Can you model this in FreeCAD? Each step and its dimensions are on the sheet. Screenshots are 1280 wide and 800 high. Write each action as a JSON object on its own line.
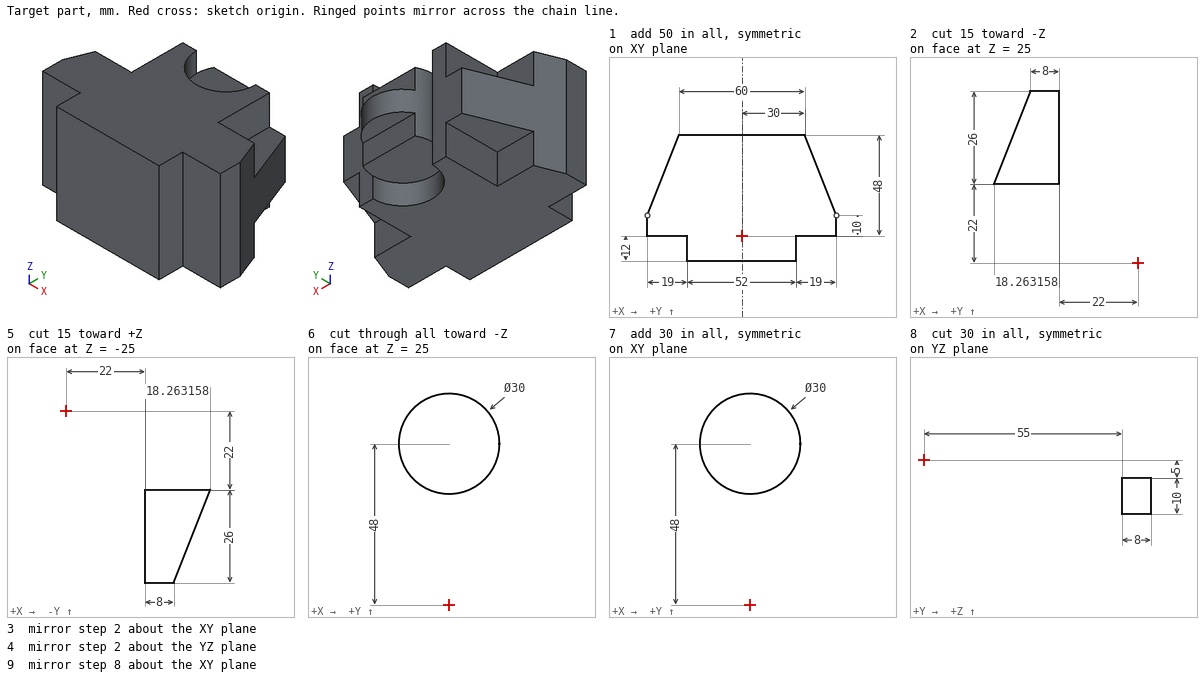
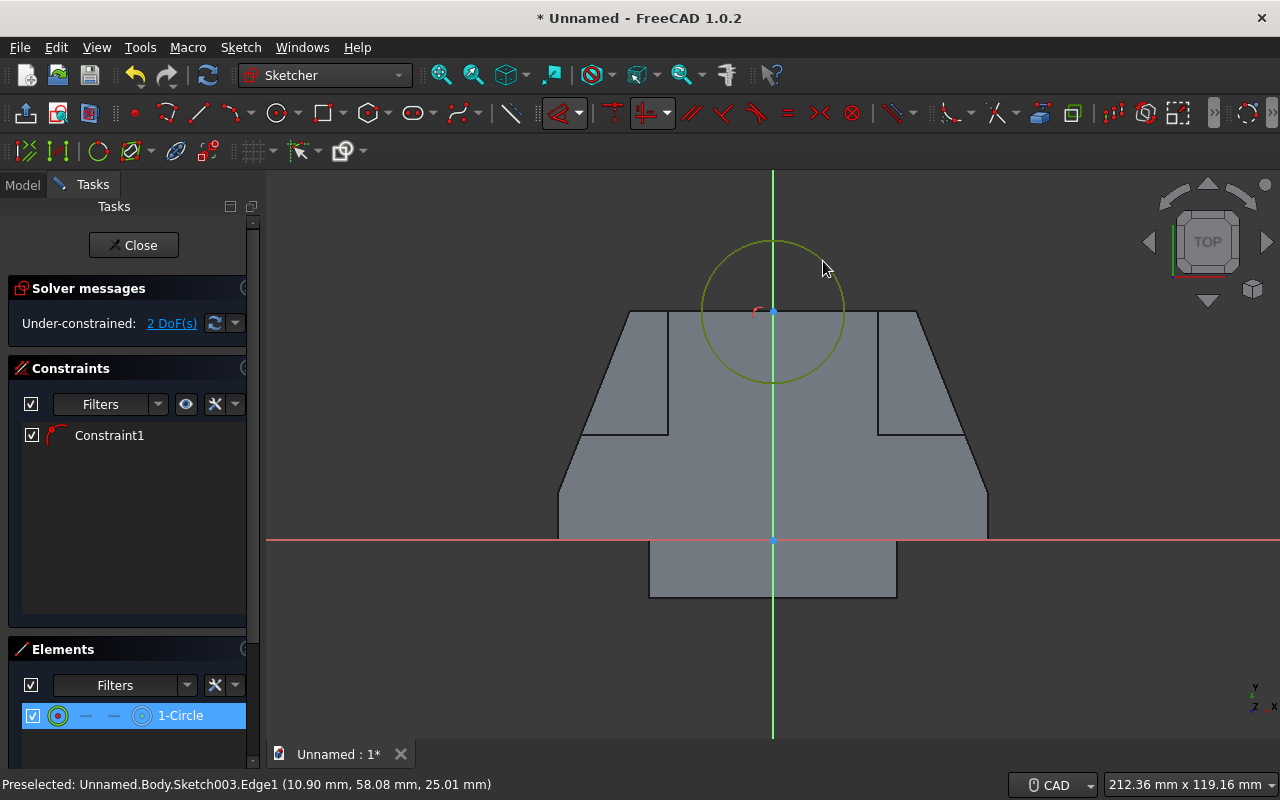
{"action": "left_click", "coordinate": [582, 114]}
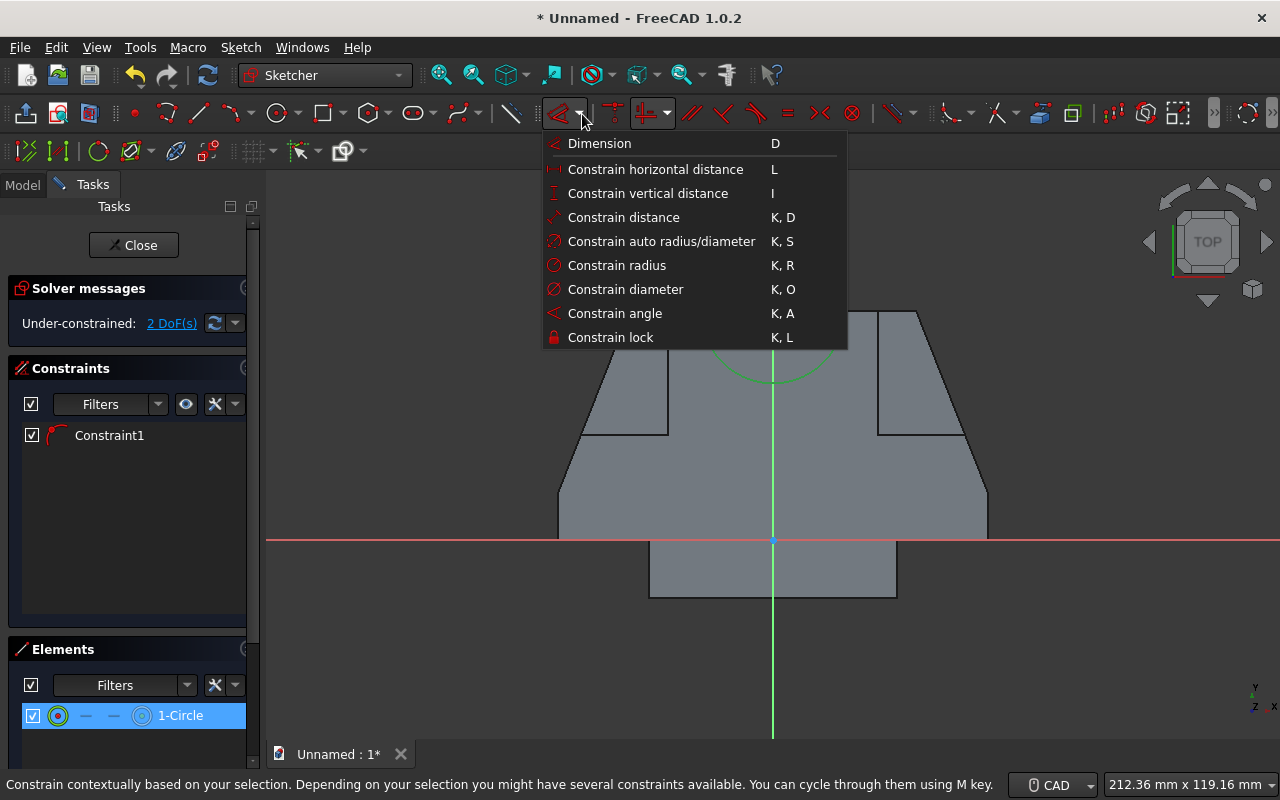
{"action": "left_click", "coordinate": [695, 289]}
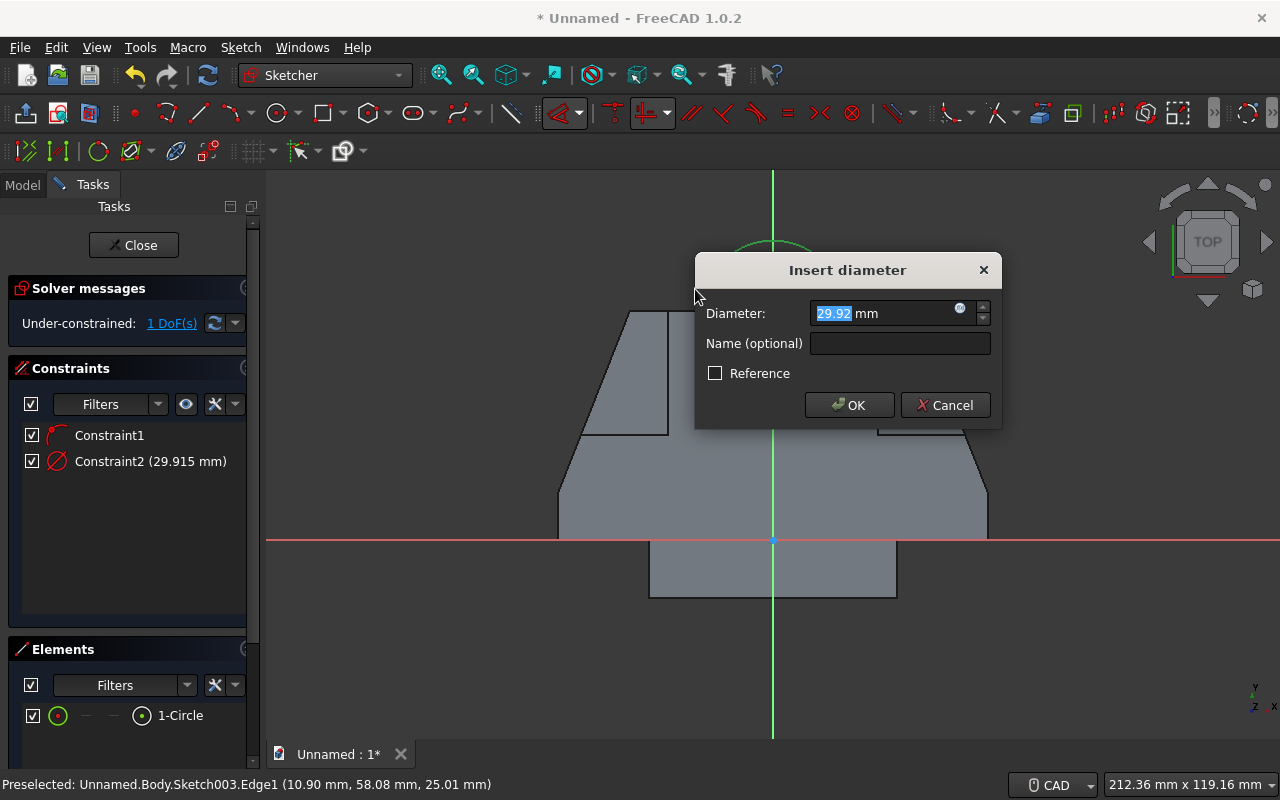
{"action": "type", "text": "30"}
{"action": "key", "text": "Return"}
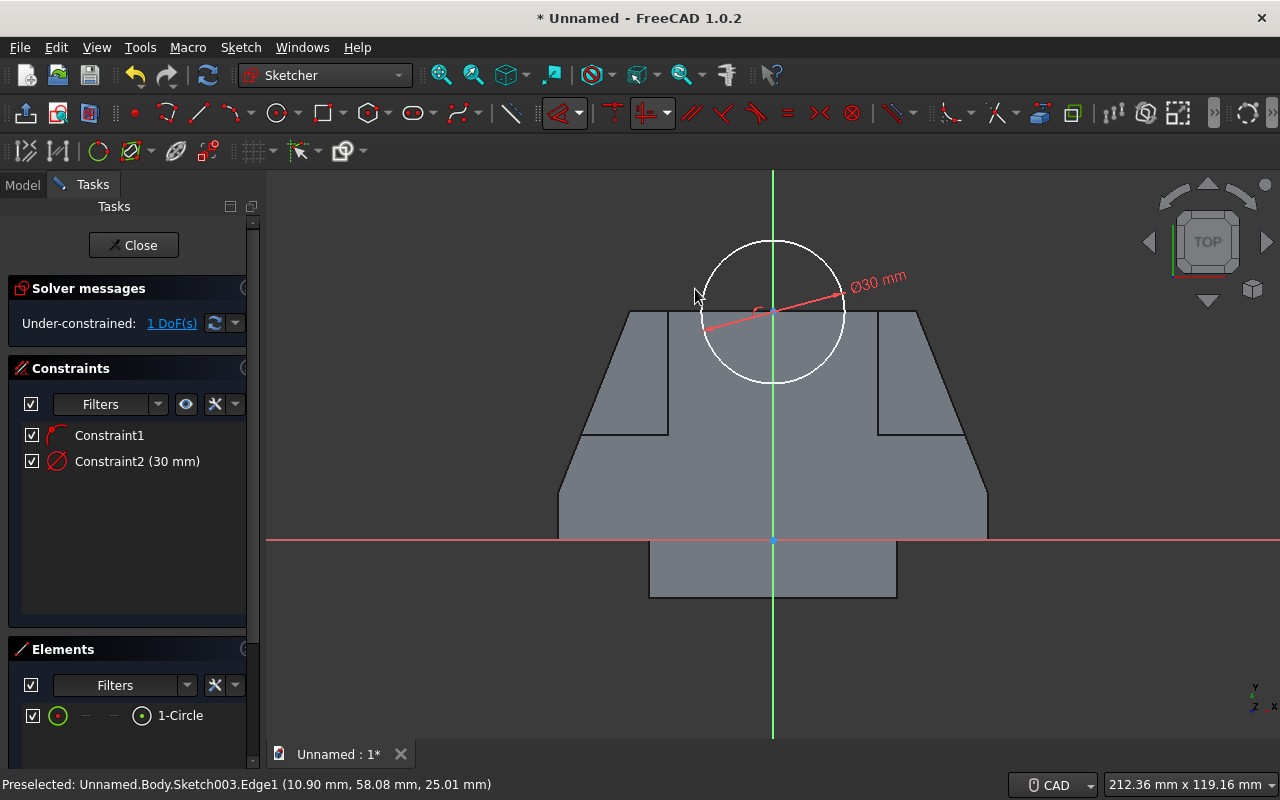
{"action": "left_click", "coordinate": [773, 312]}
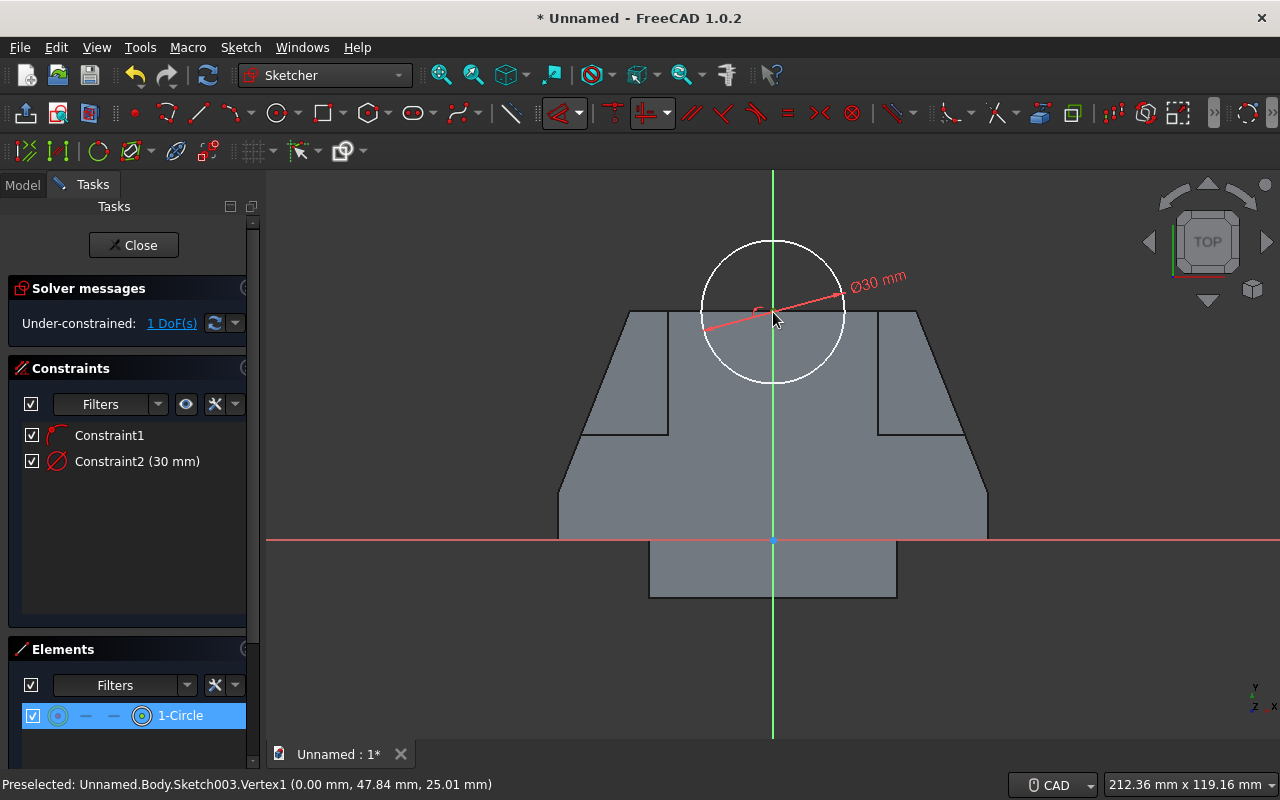
{"action": "left_click", "coordinate": [582, 114]}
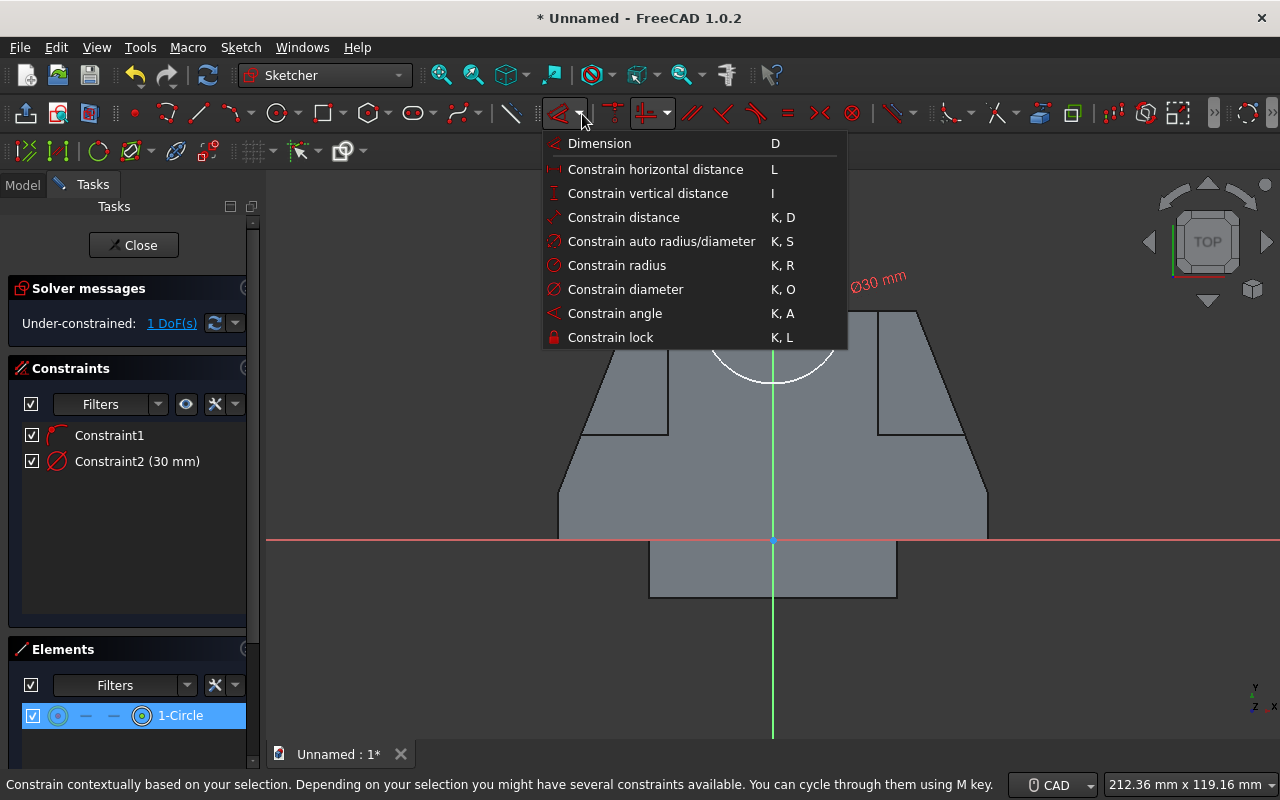
{"action": "left_click", "coordinate": [695, 193]}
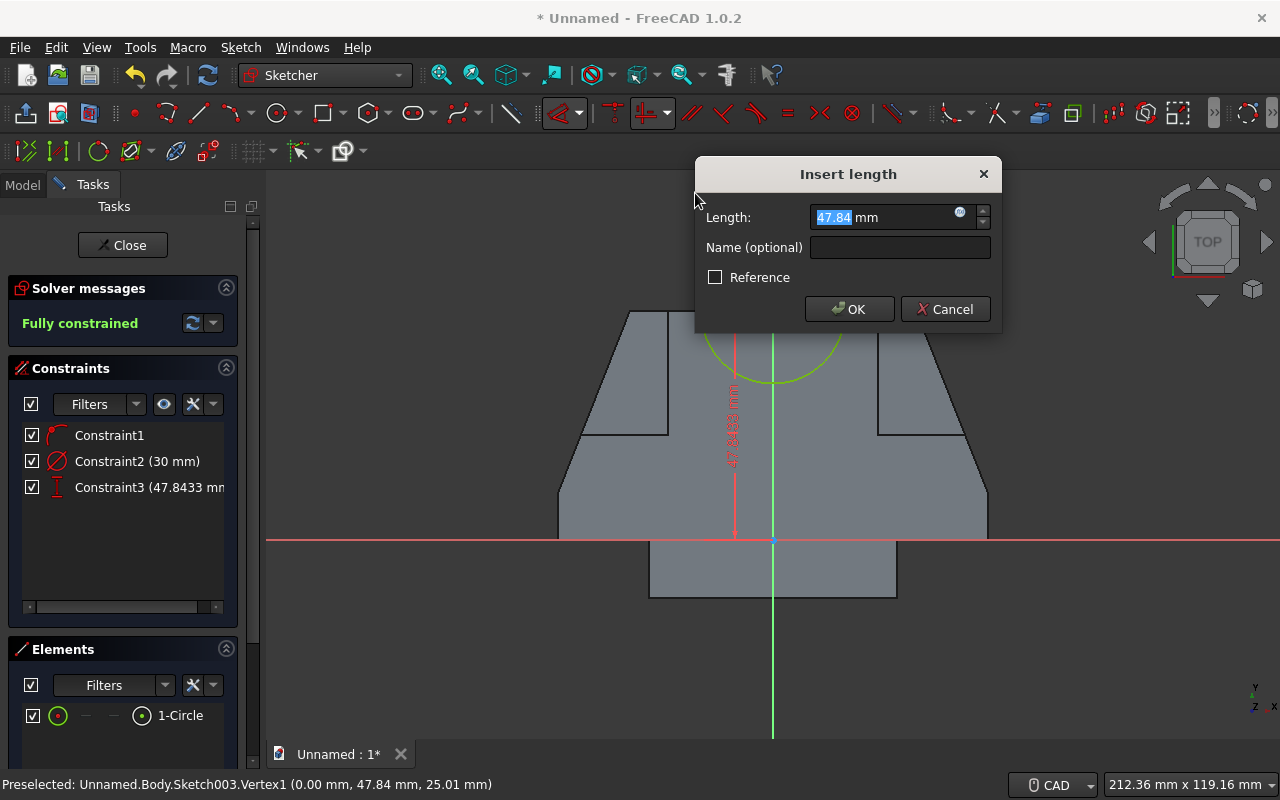
{"action": "type", "text": "48"}
{"action": "key", "text": "Return"}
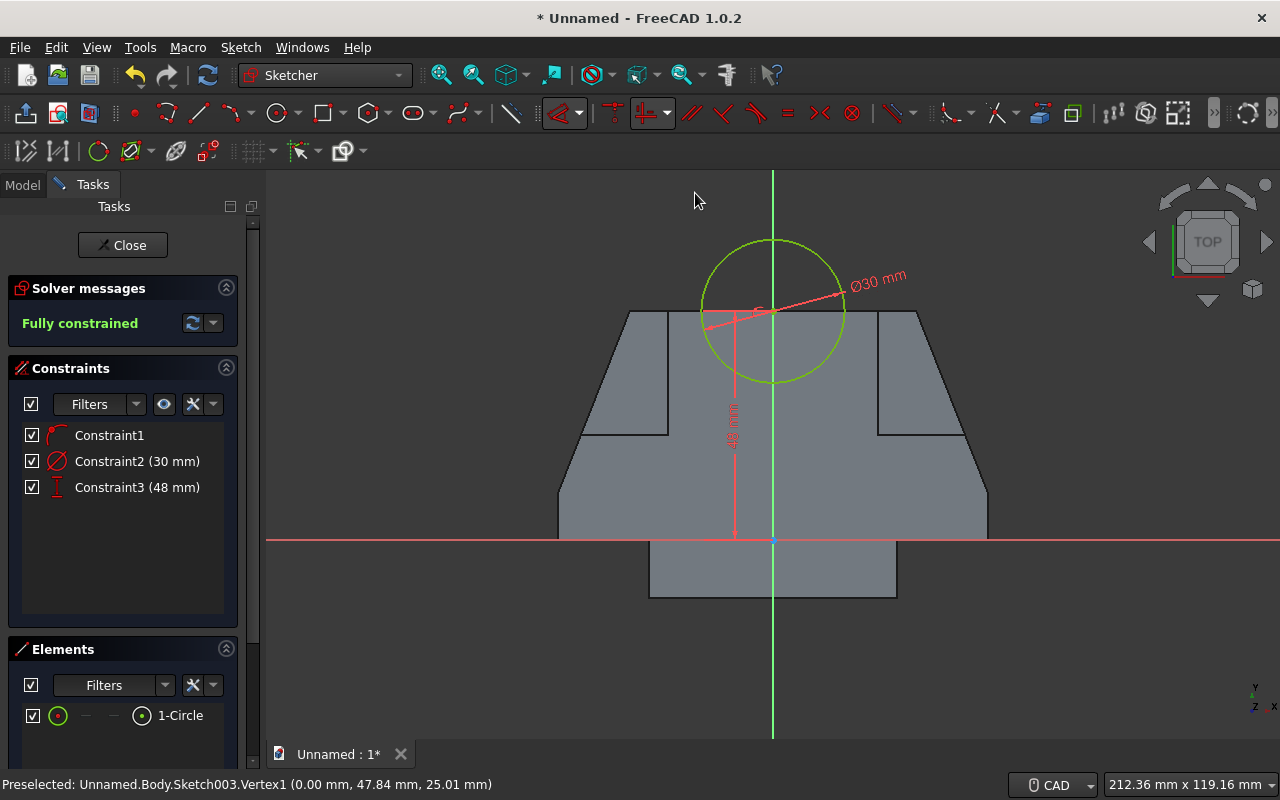
{"action": "left_click", "coordinate": [123, 245]}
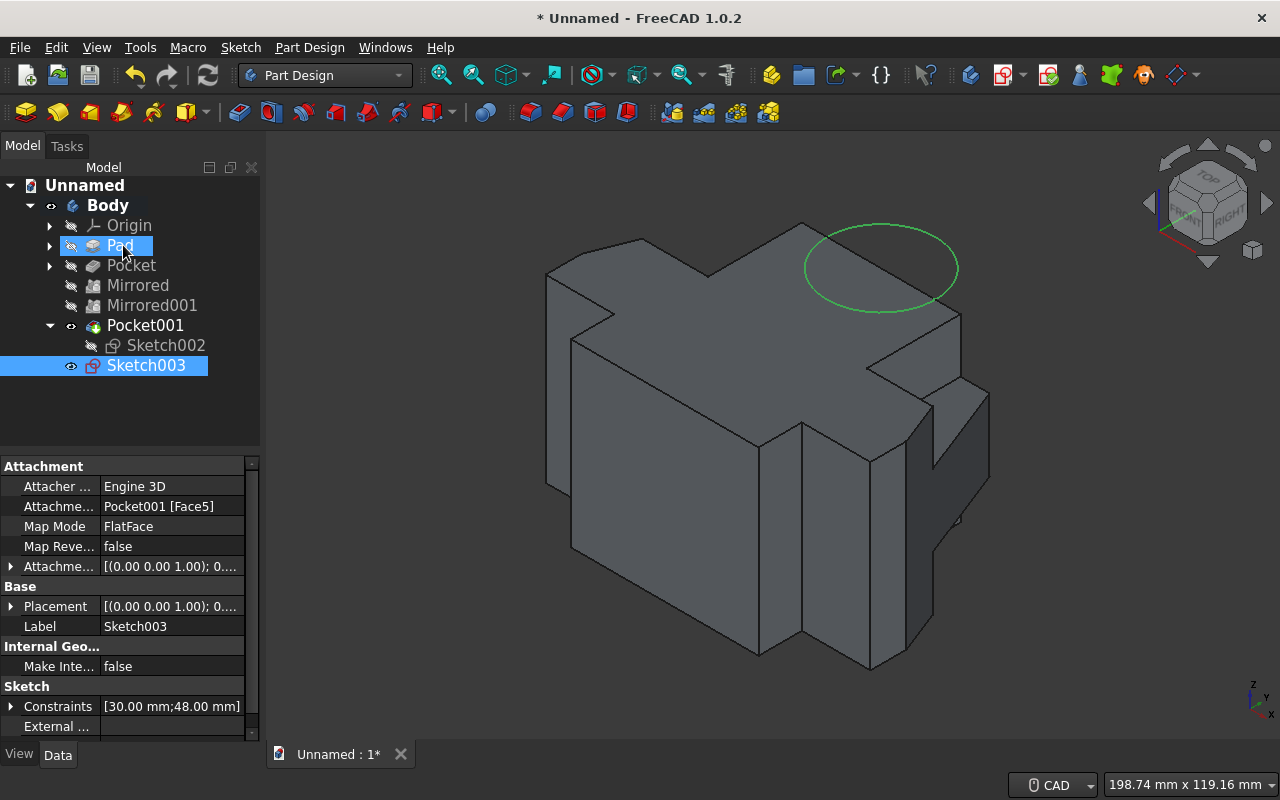
{"action": "left_click", "coordinate": [240, 112]}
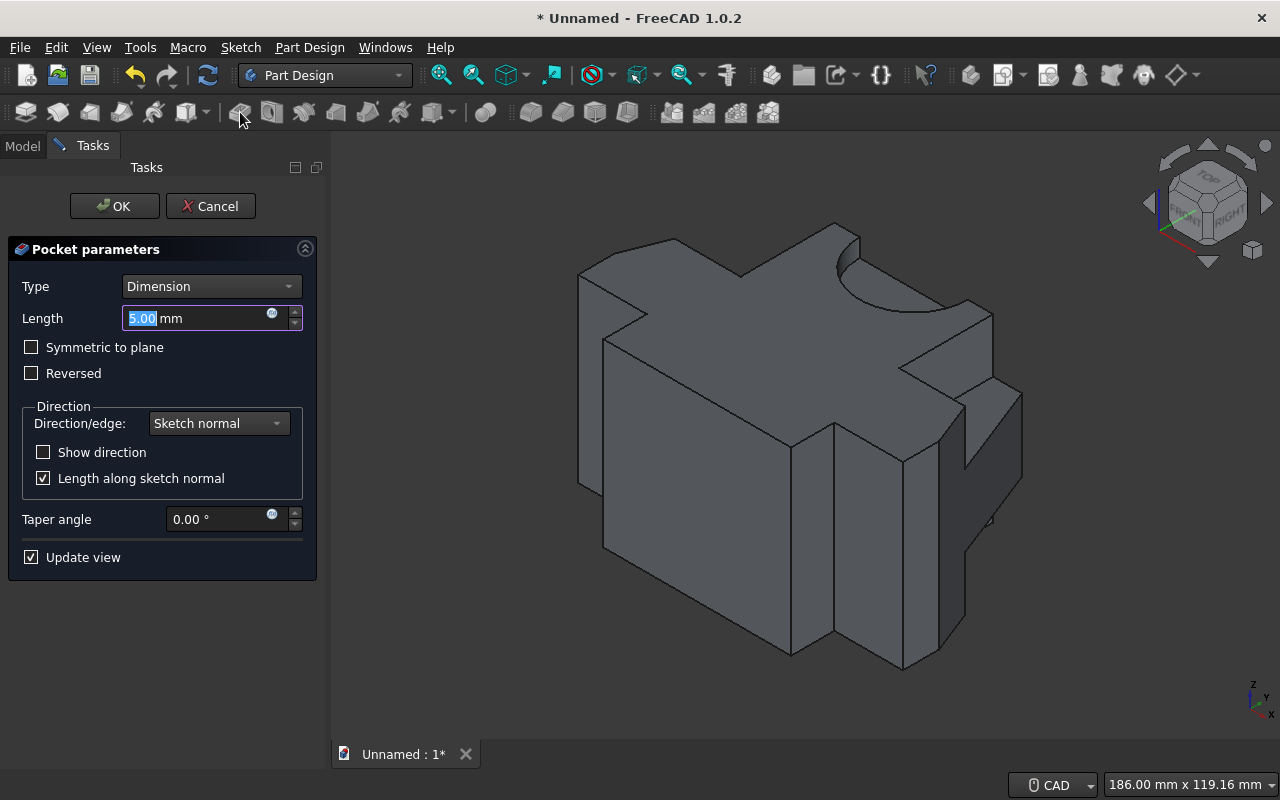
{"action": "left_click", "coordinate": [212, 286]}